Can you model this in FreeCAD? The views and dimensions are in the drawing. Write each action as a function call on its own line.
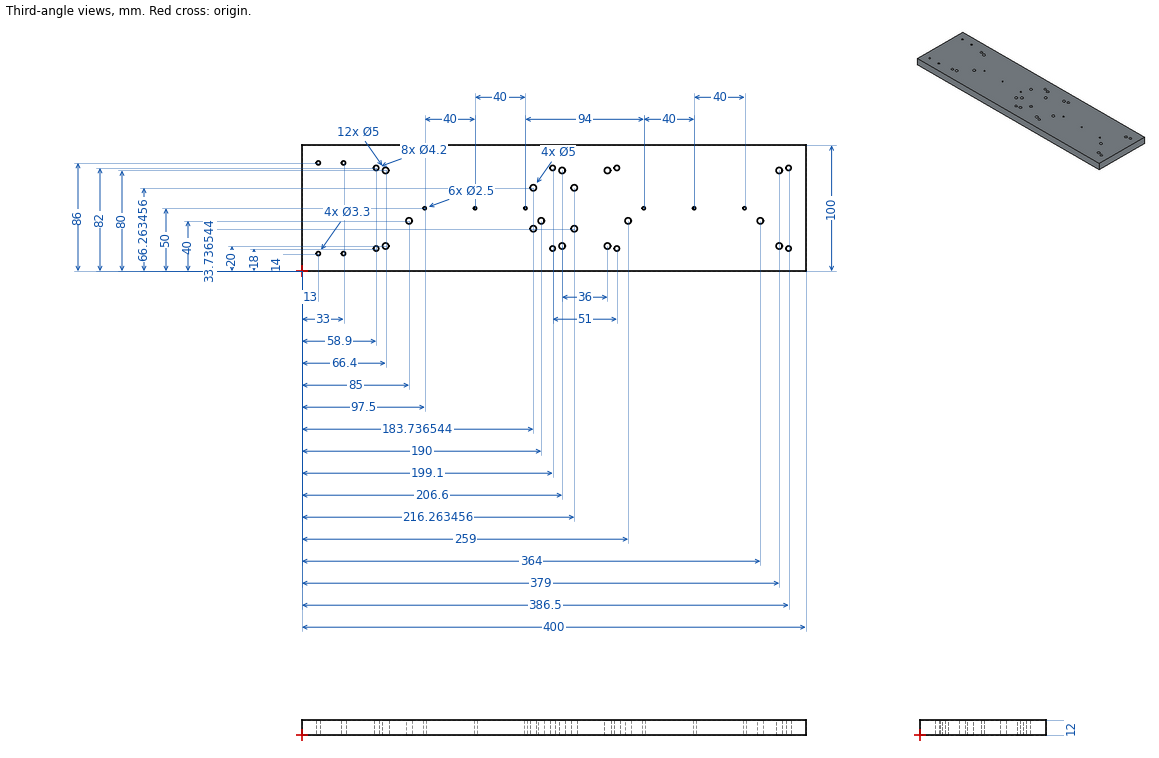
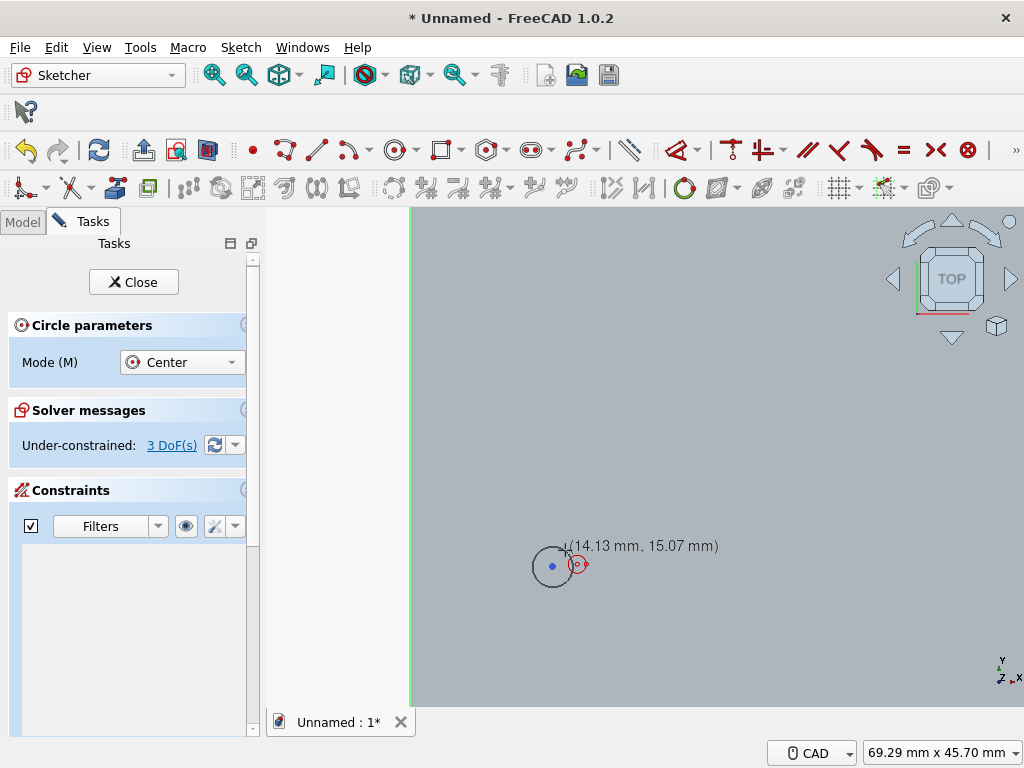
scroll(566, 552, down, 6)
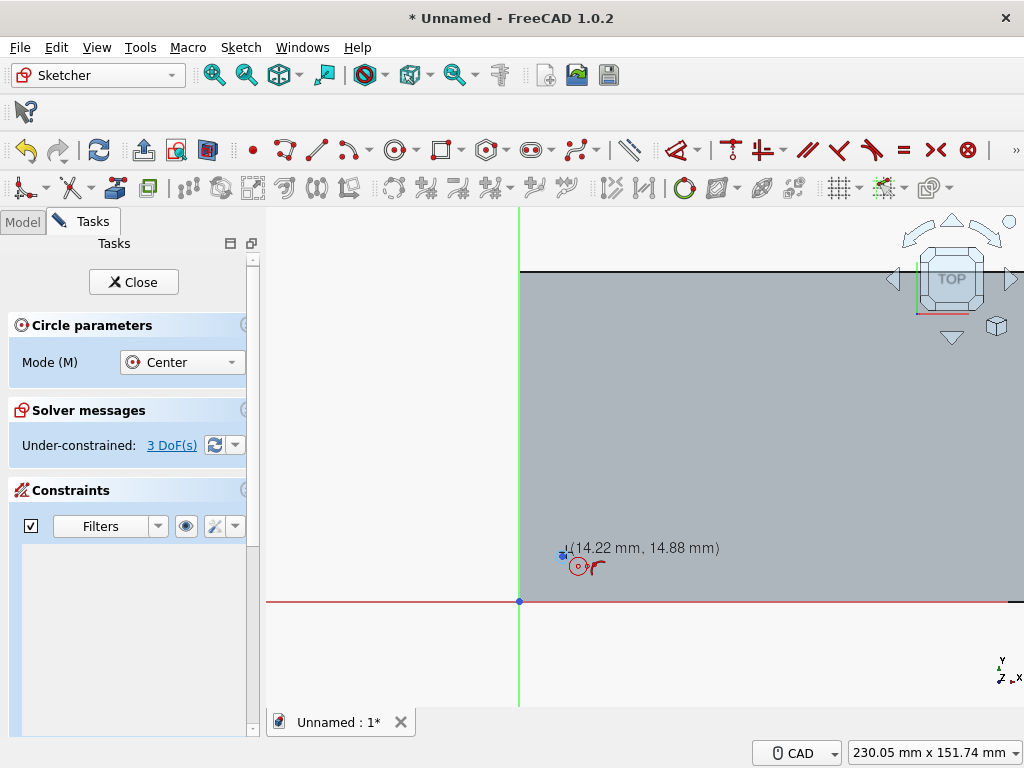
scroll(562, 318, up, 8)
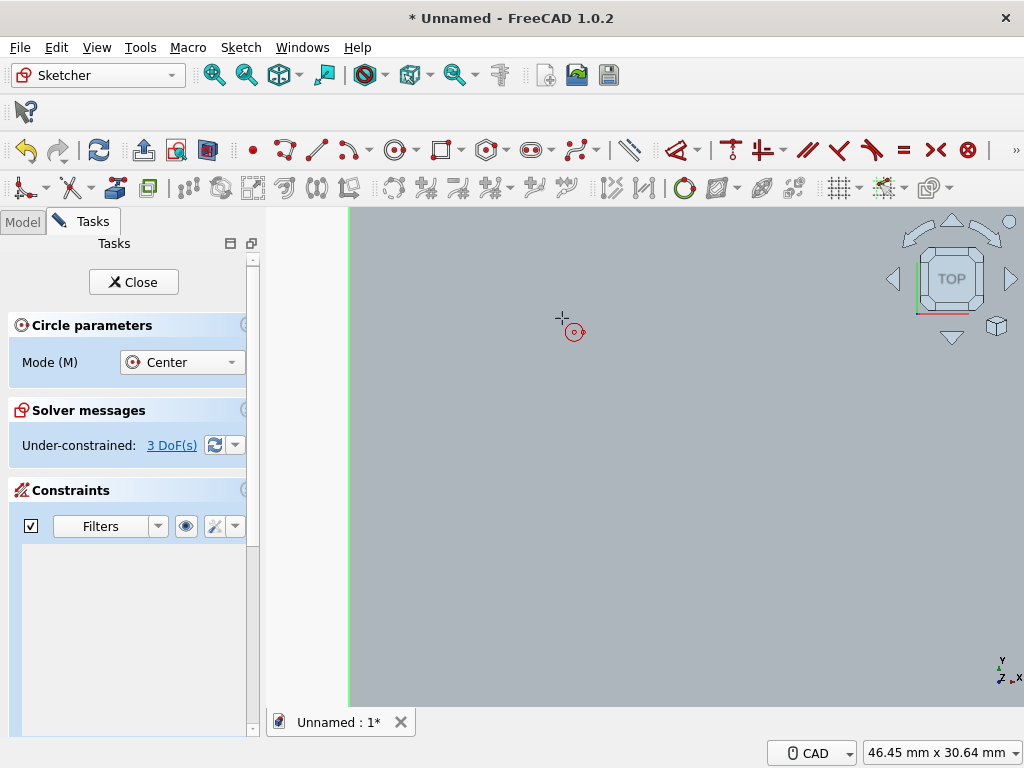
scroll(562, 318, down, 8)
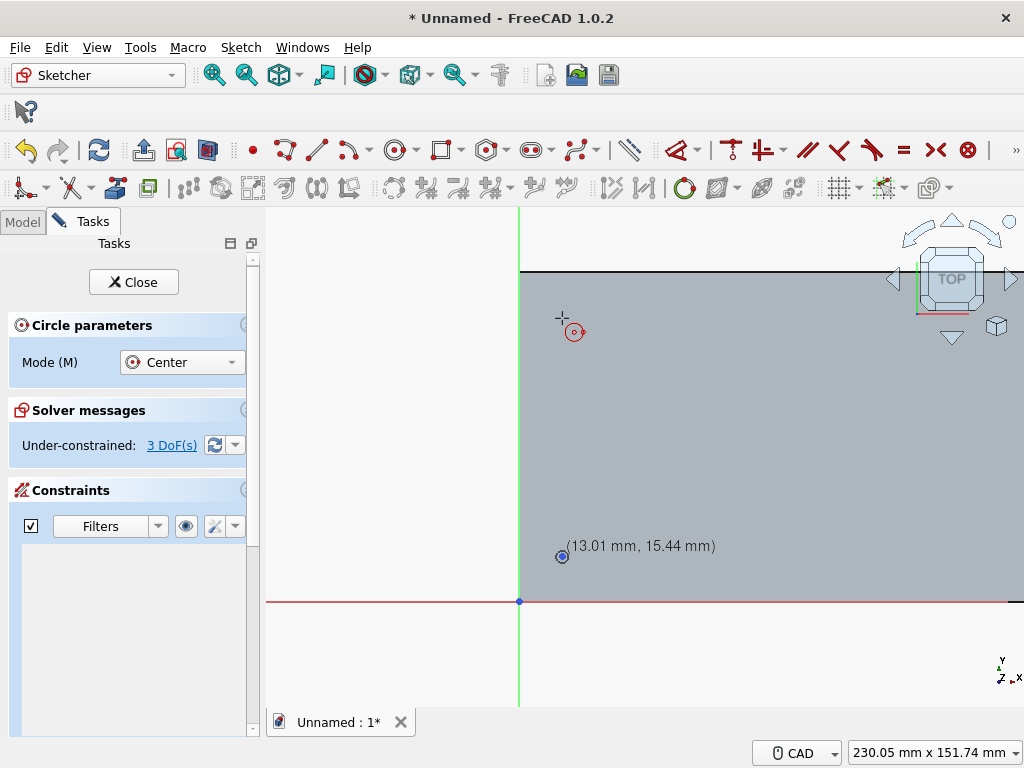
click(562, 318)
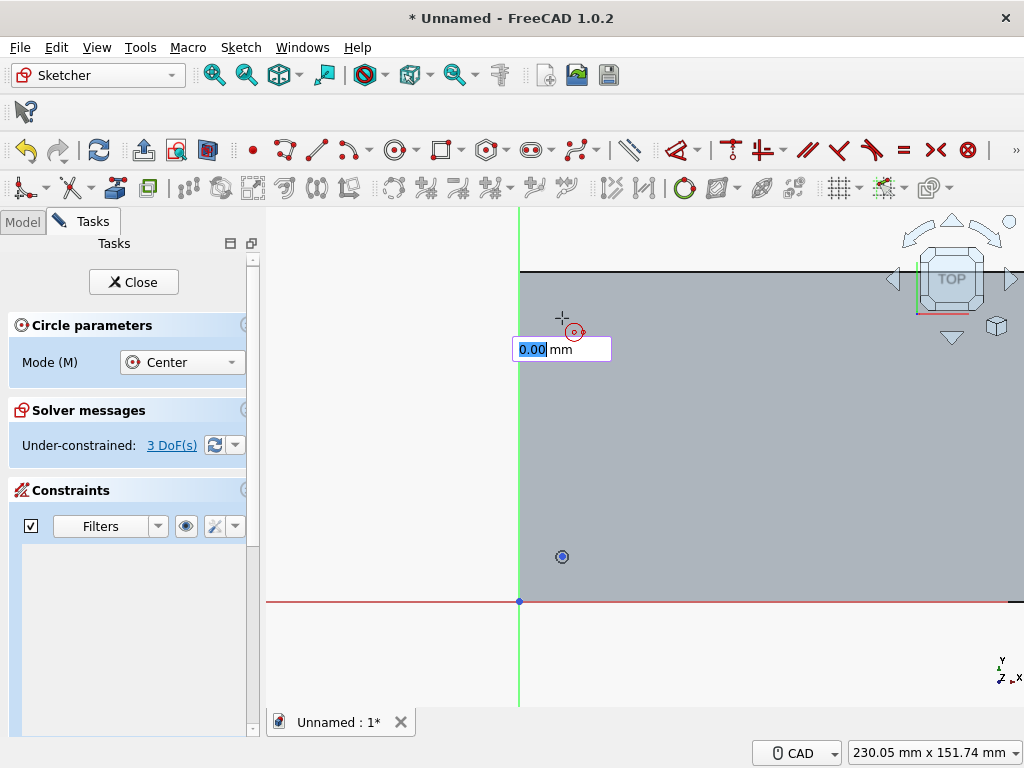
scroll(566, 315, up, 6)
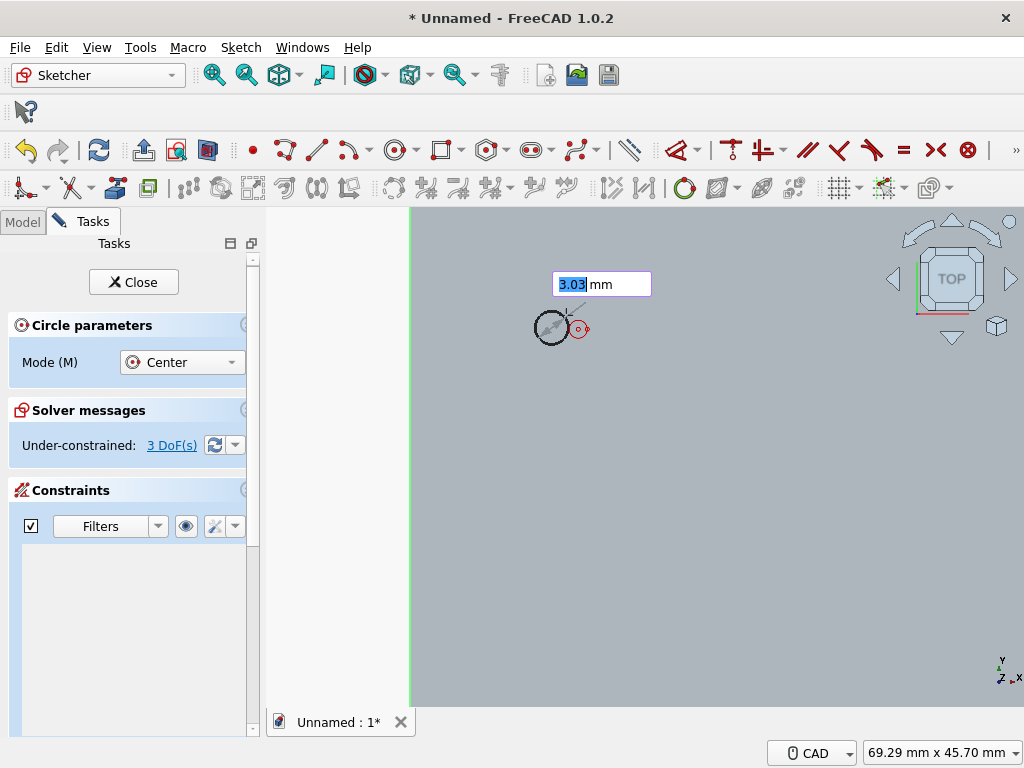
click(565, 313)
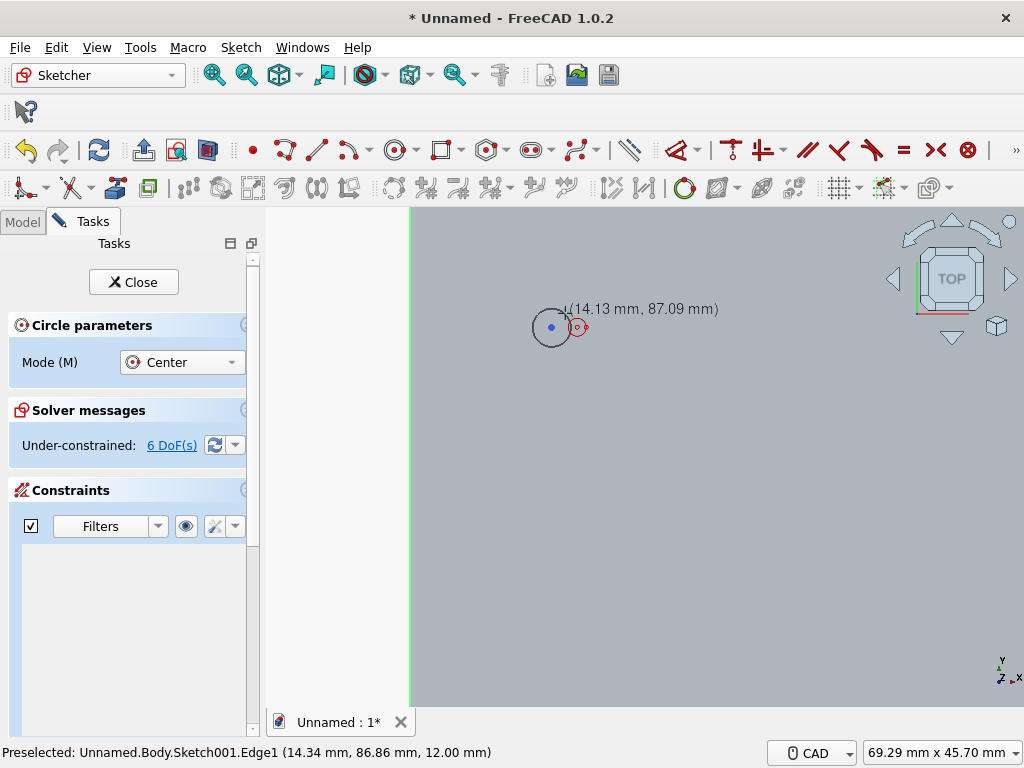
scroll(771, 326, up, 2)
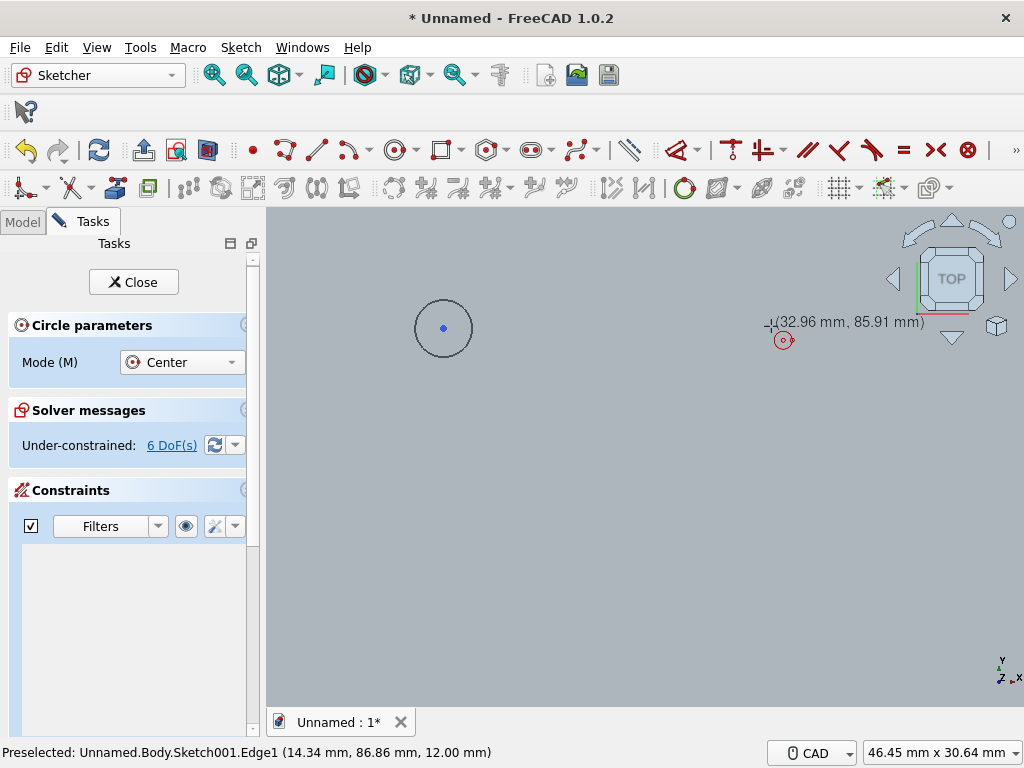
scroll(592, 316, down, 8)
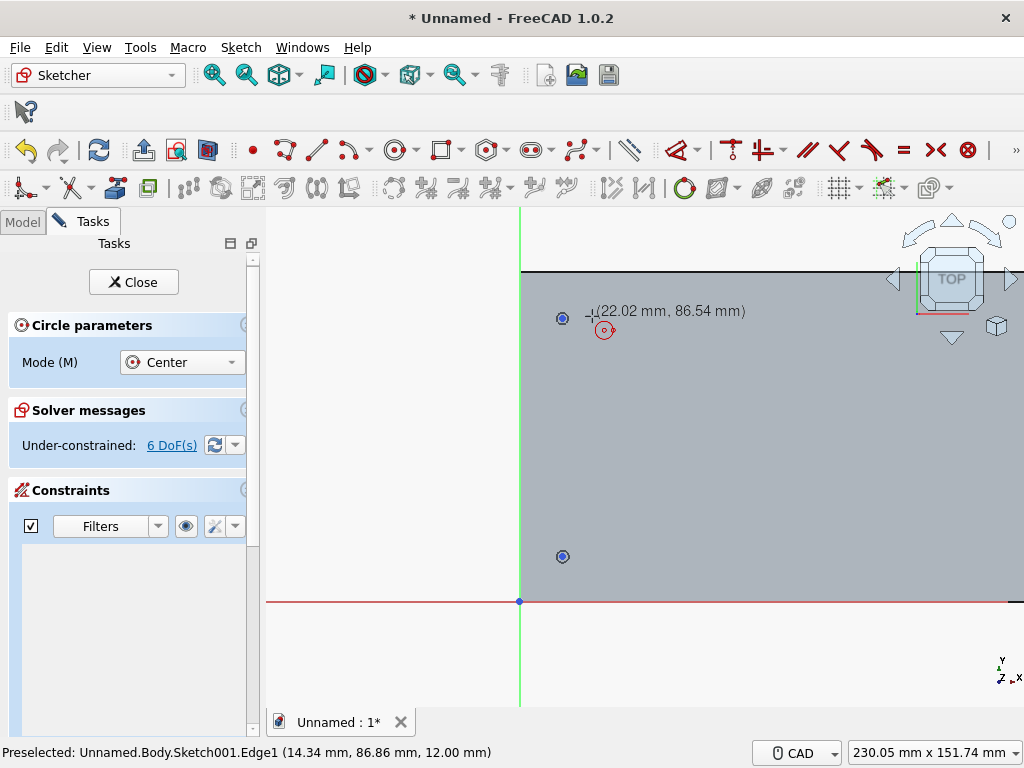
click(629, 318)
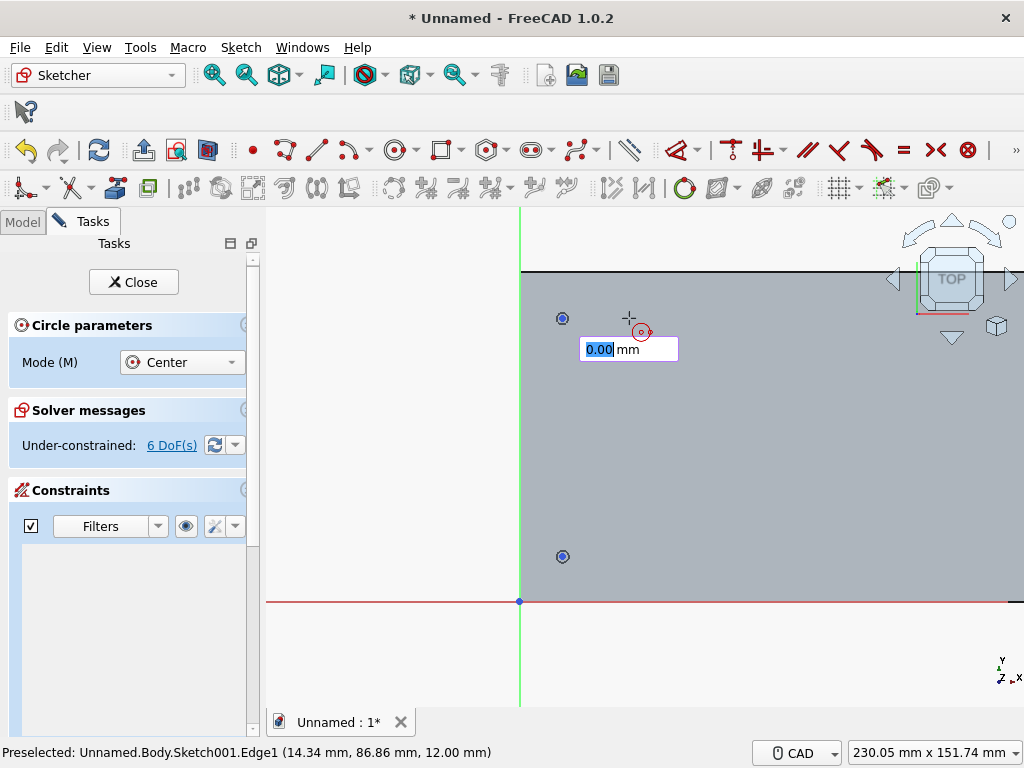
scroll(632, 314, up, 6)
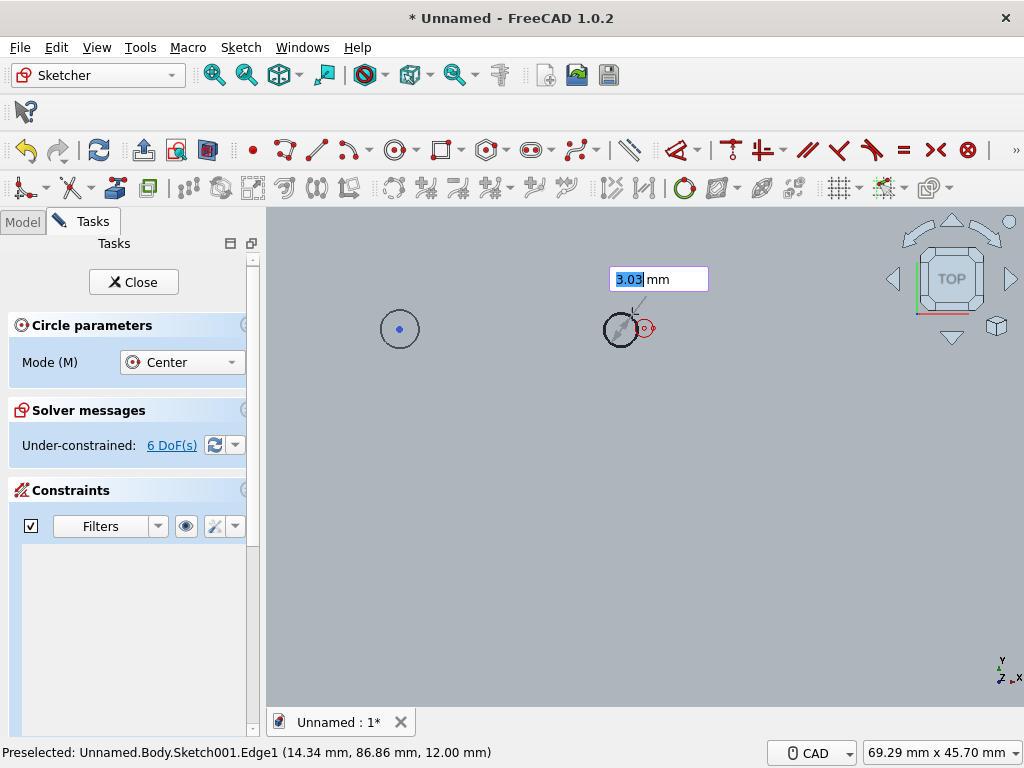
click(632, 315)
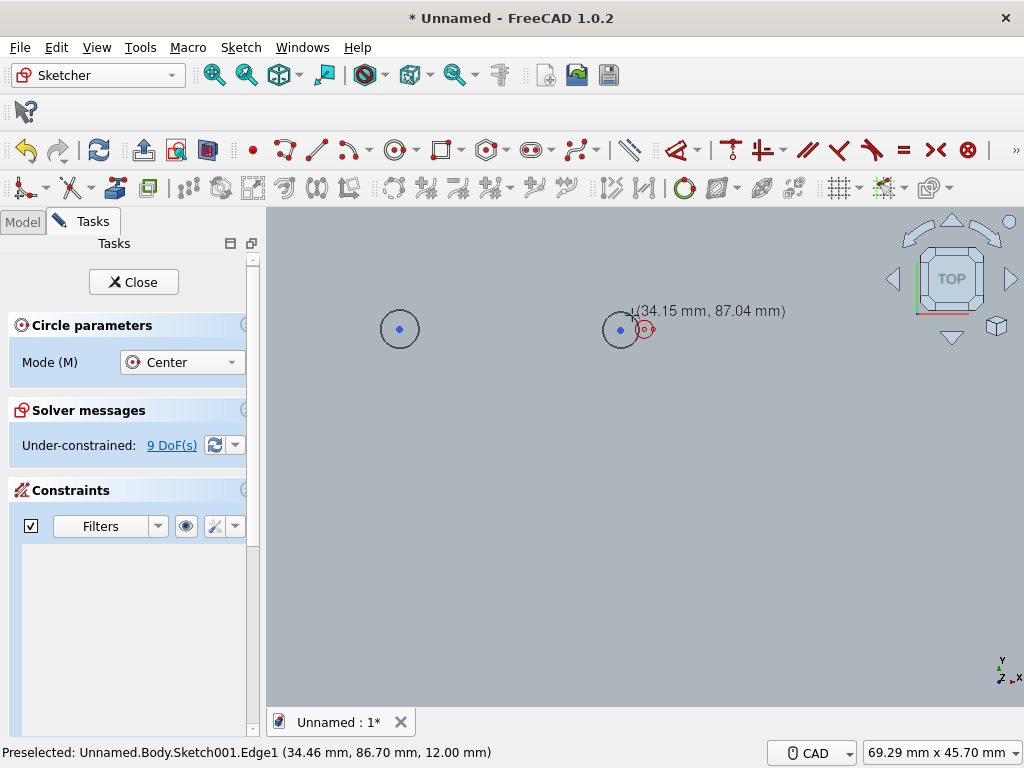
scroll(632, 314, down, 6)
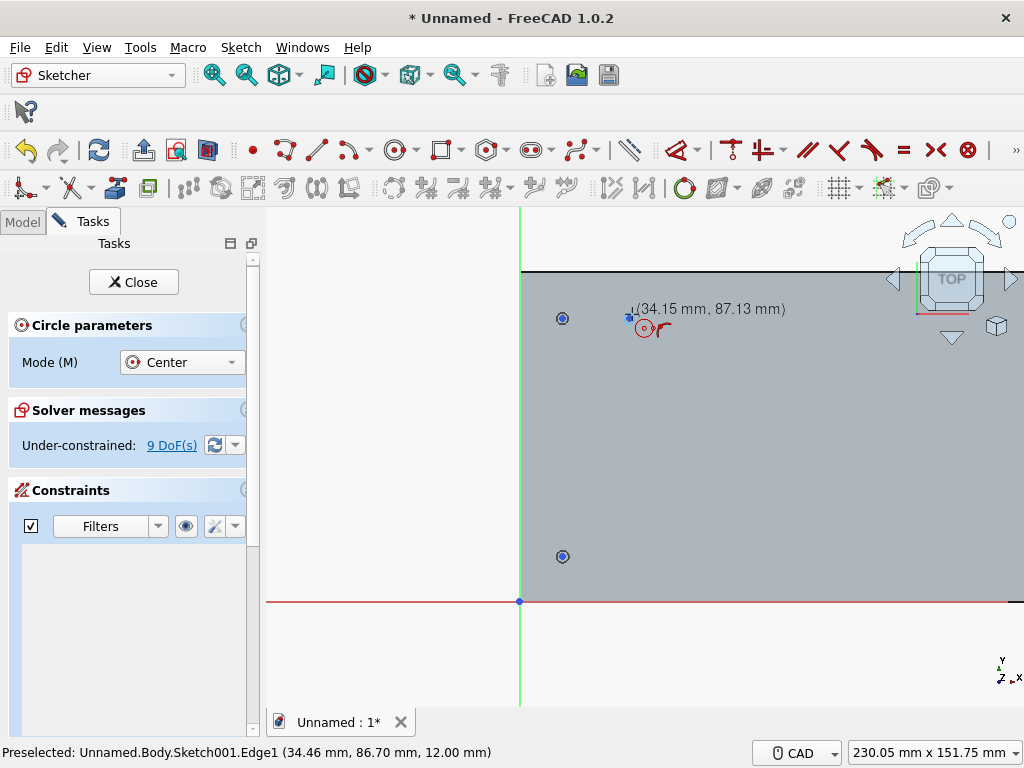
scroll(629, 555, up, 8)